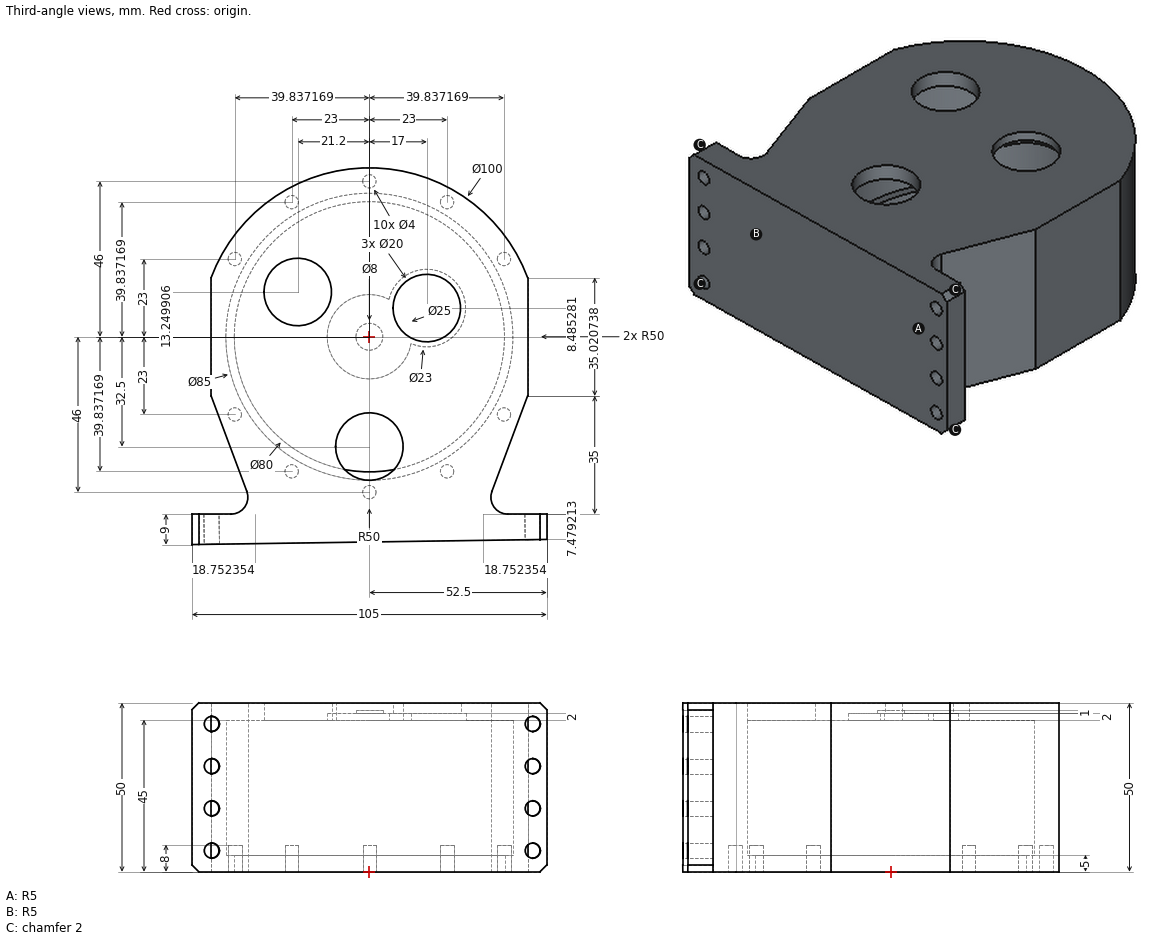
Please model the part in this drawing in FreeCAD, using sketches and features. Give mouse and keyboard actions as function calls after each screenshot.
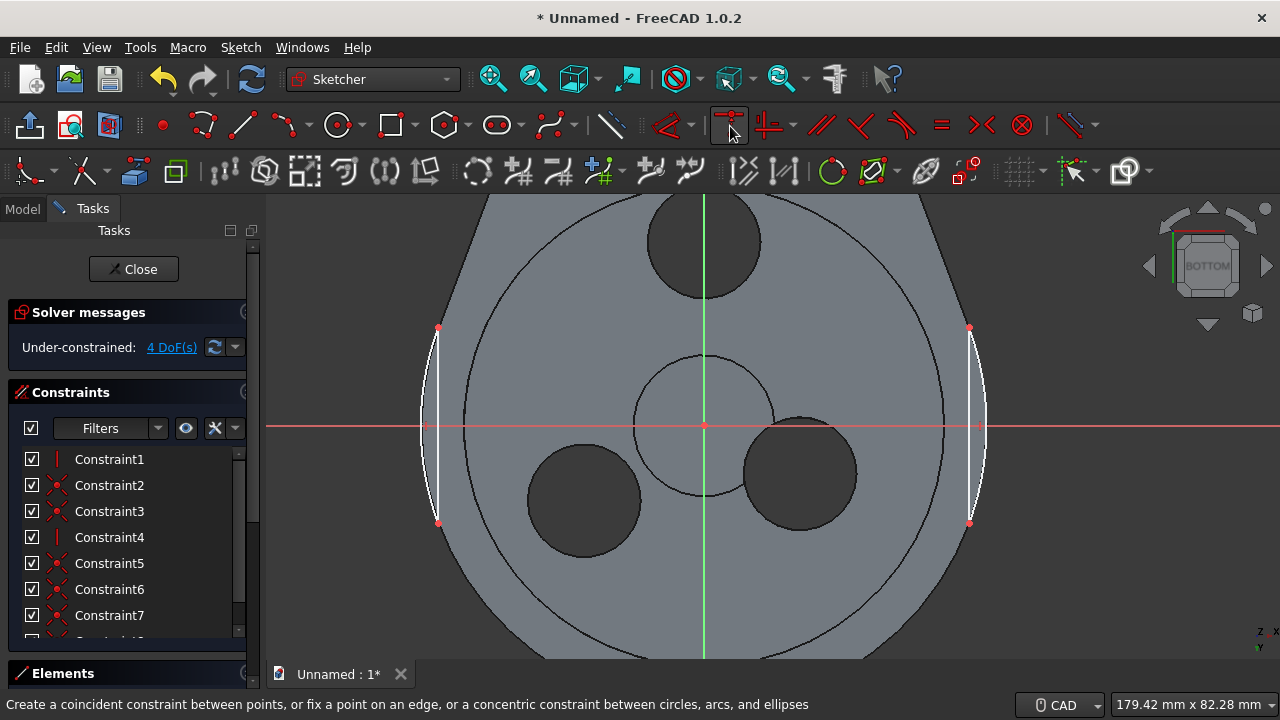
click(984, 466)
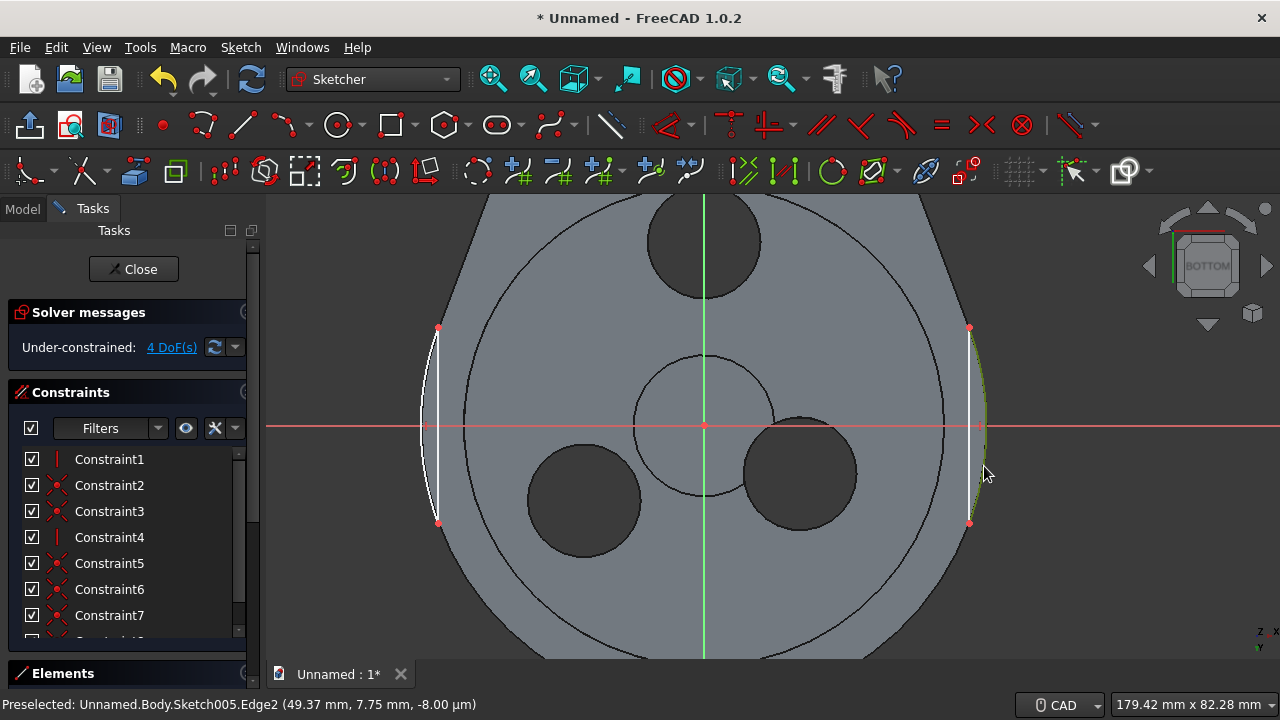
click(424, 386)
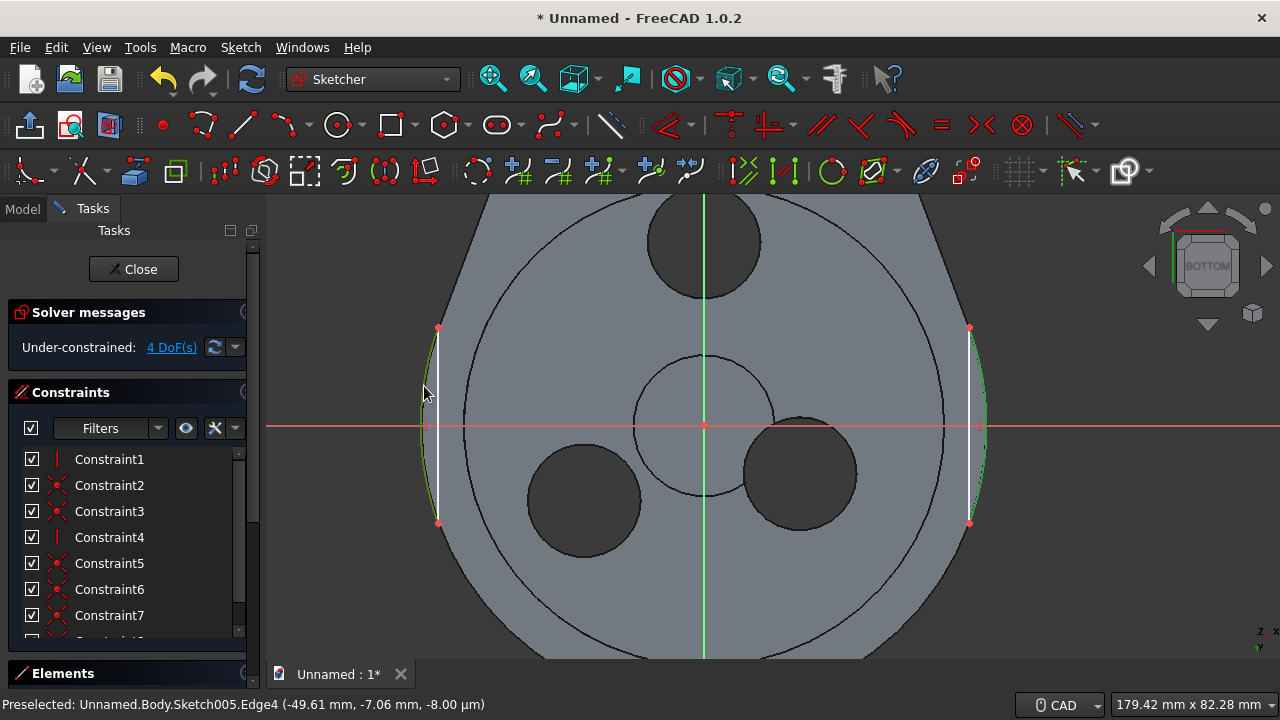
click(942, 126)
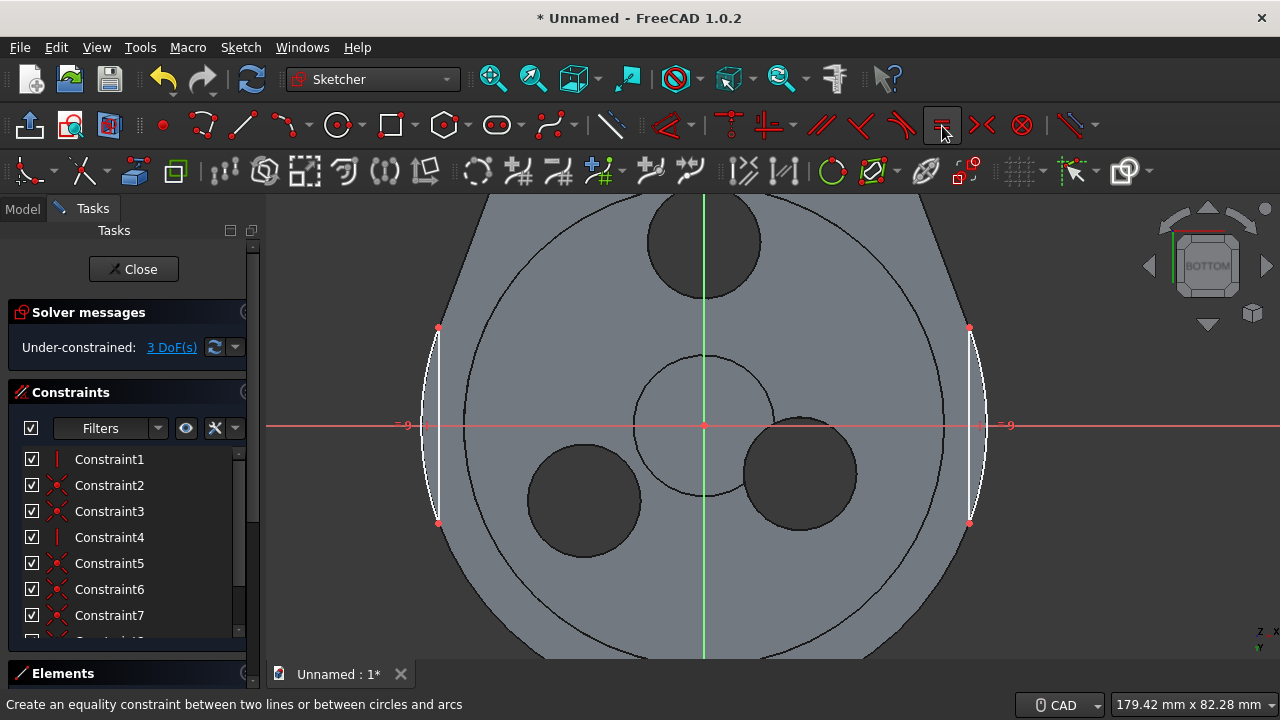
click(666, 126)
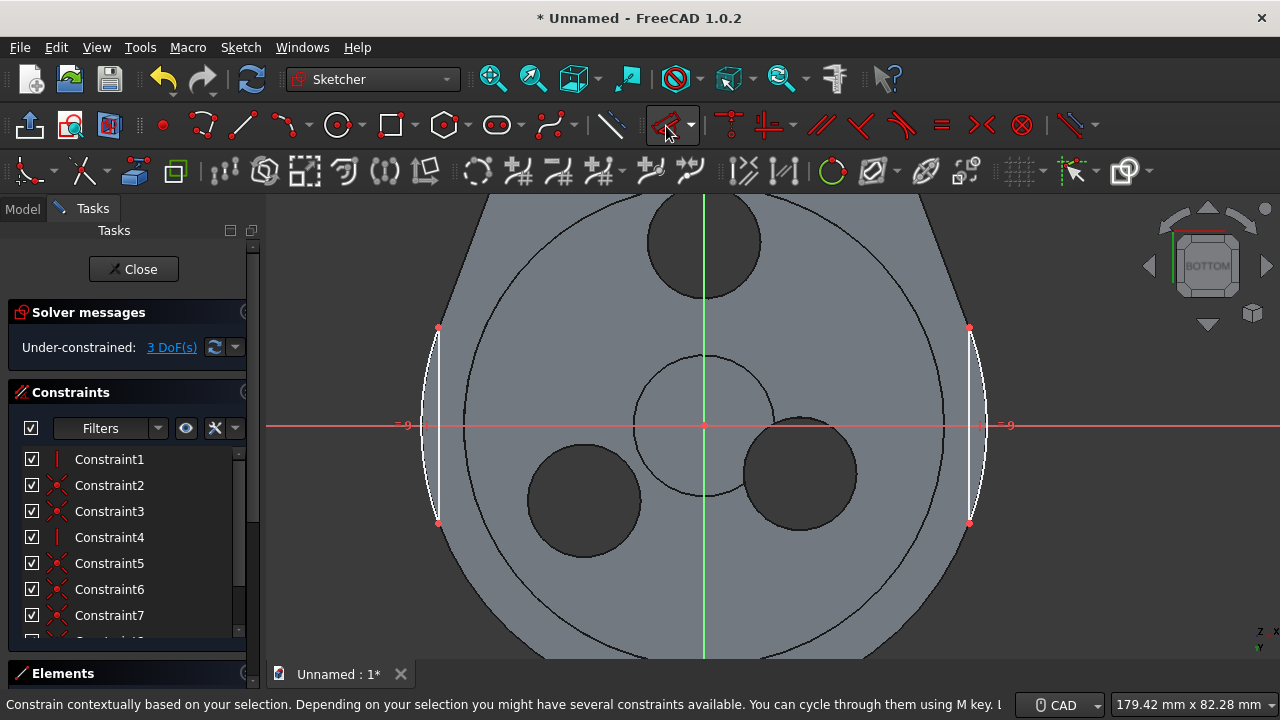
click(984, 466)
click(1016, 471)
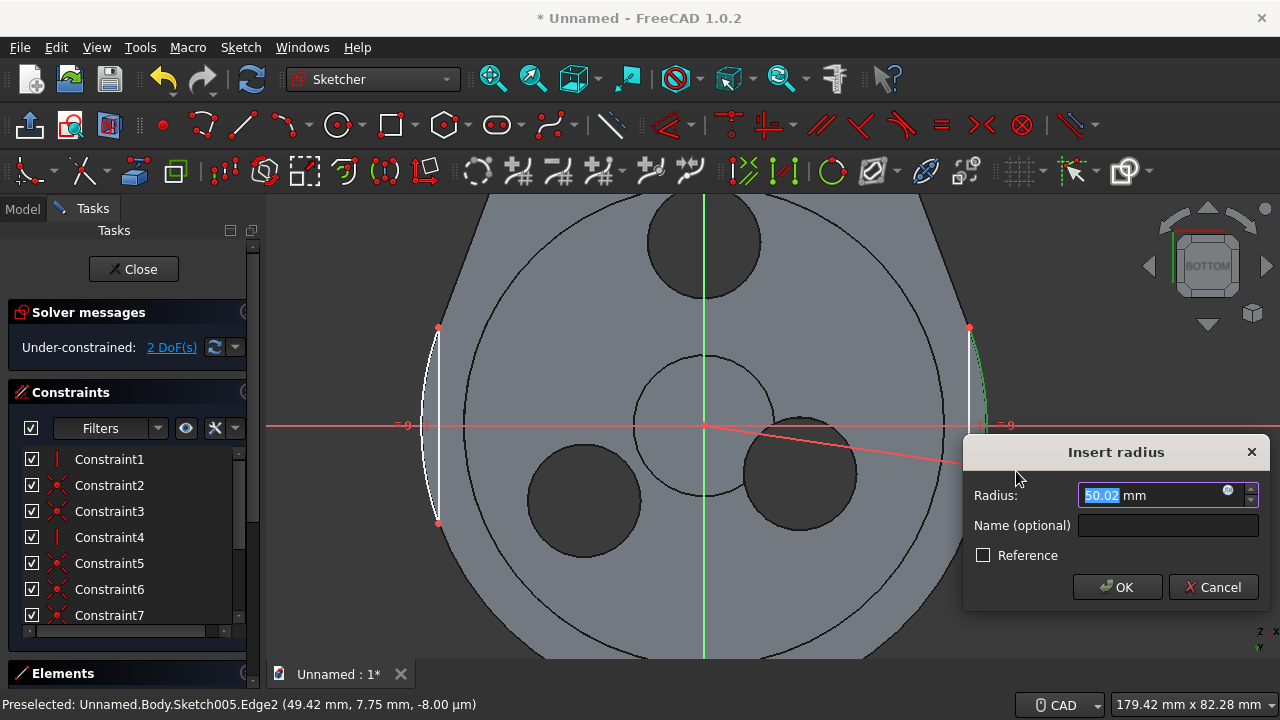
text(50)
key(Return)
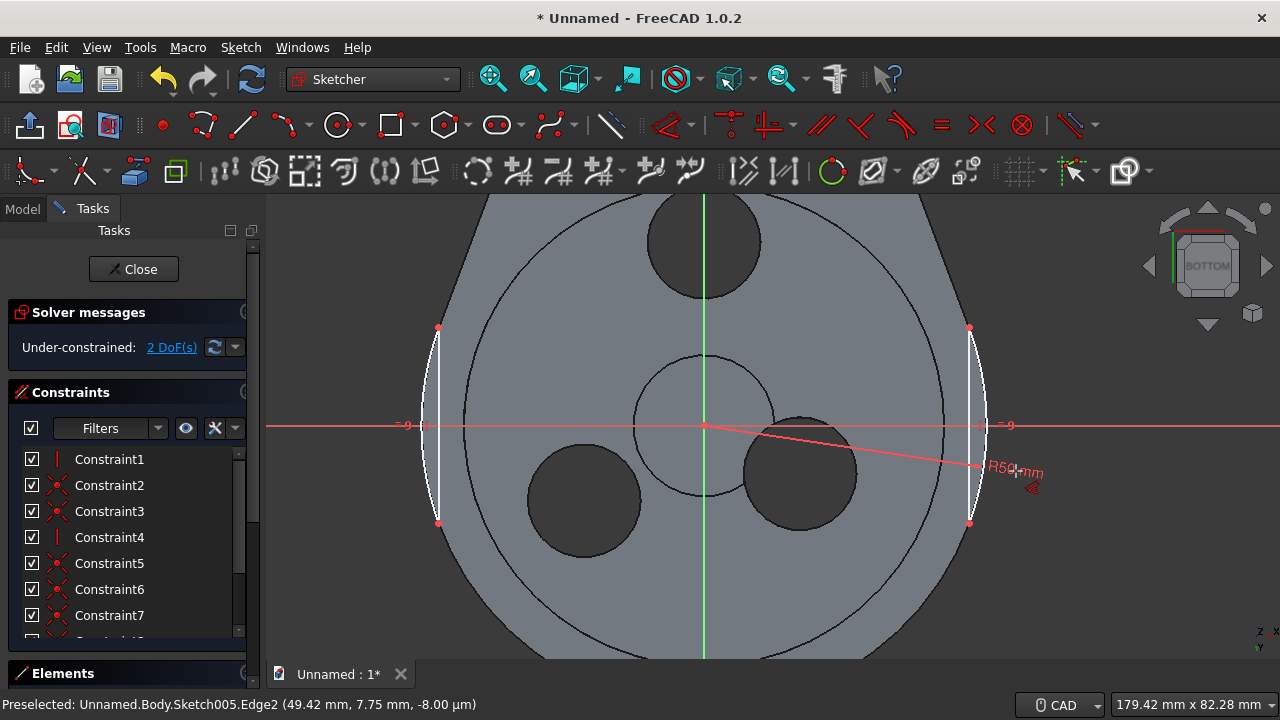
click(969, 387)
click(1003, 381)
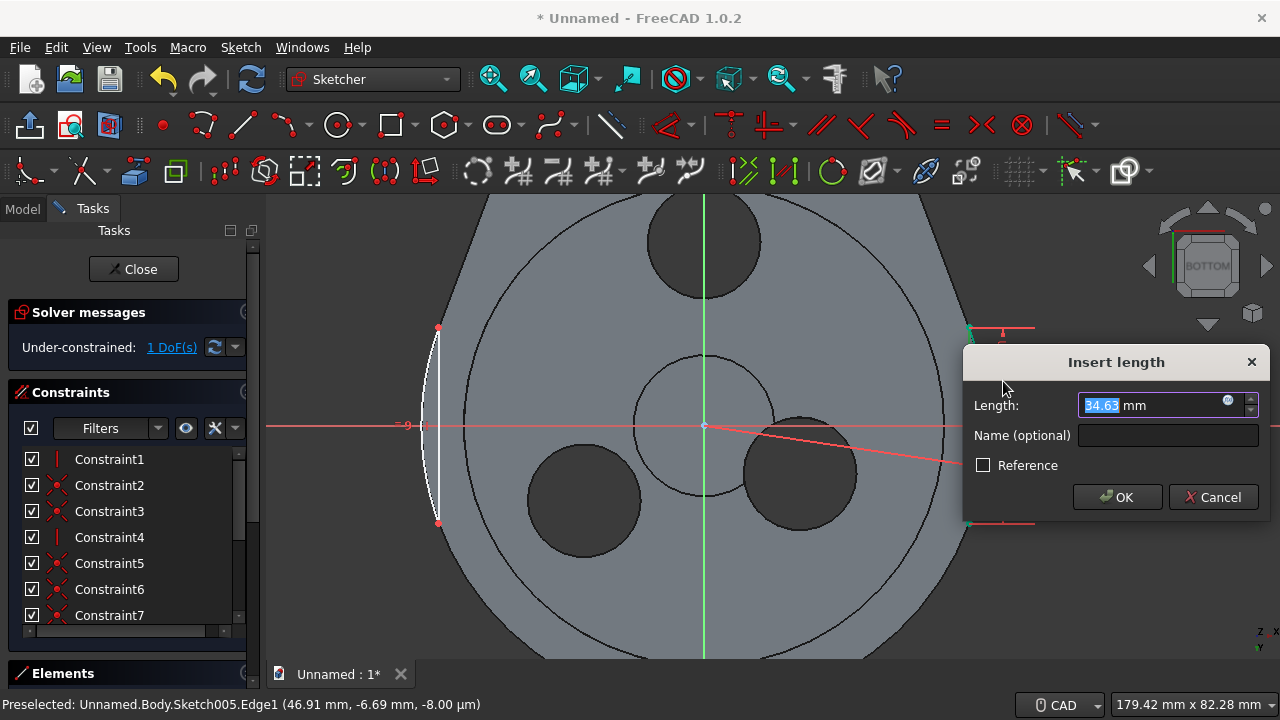
text(35.020738)
key(Return)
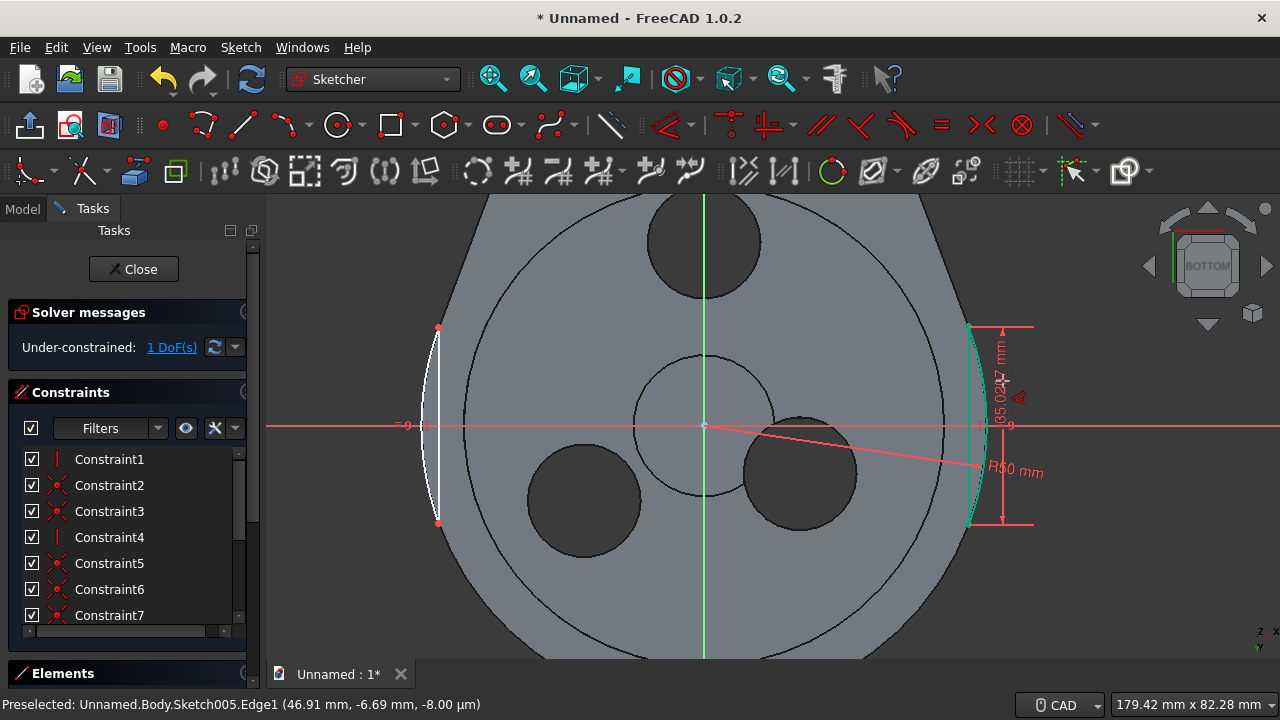
click(439, 465)
click(405, 381)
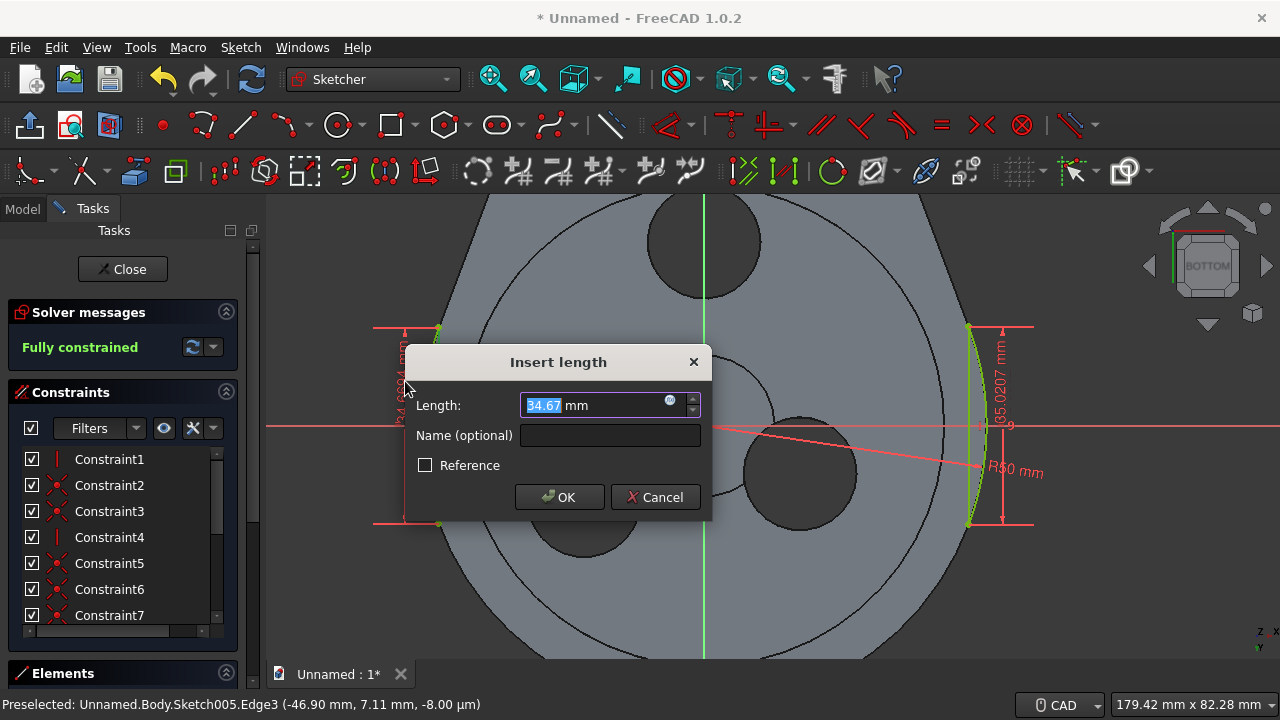
text(35.020738)
key(Return)
key(Escape)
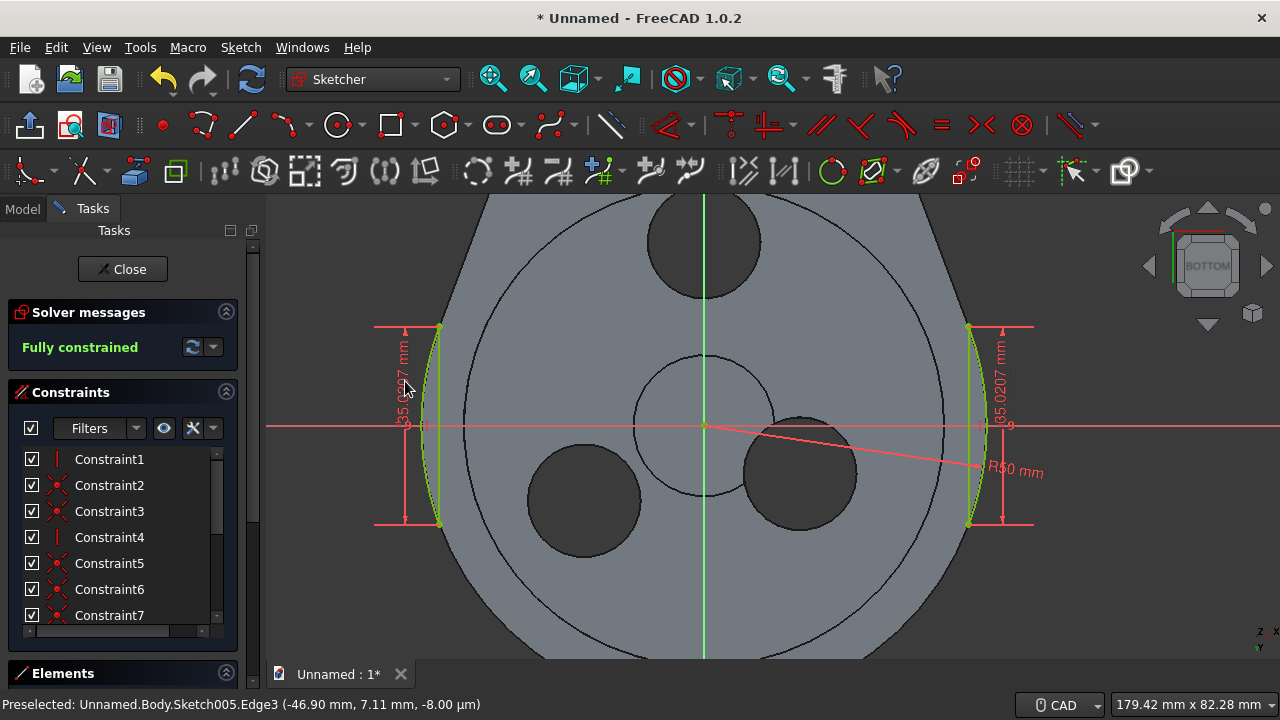
click(123, 269)